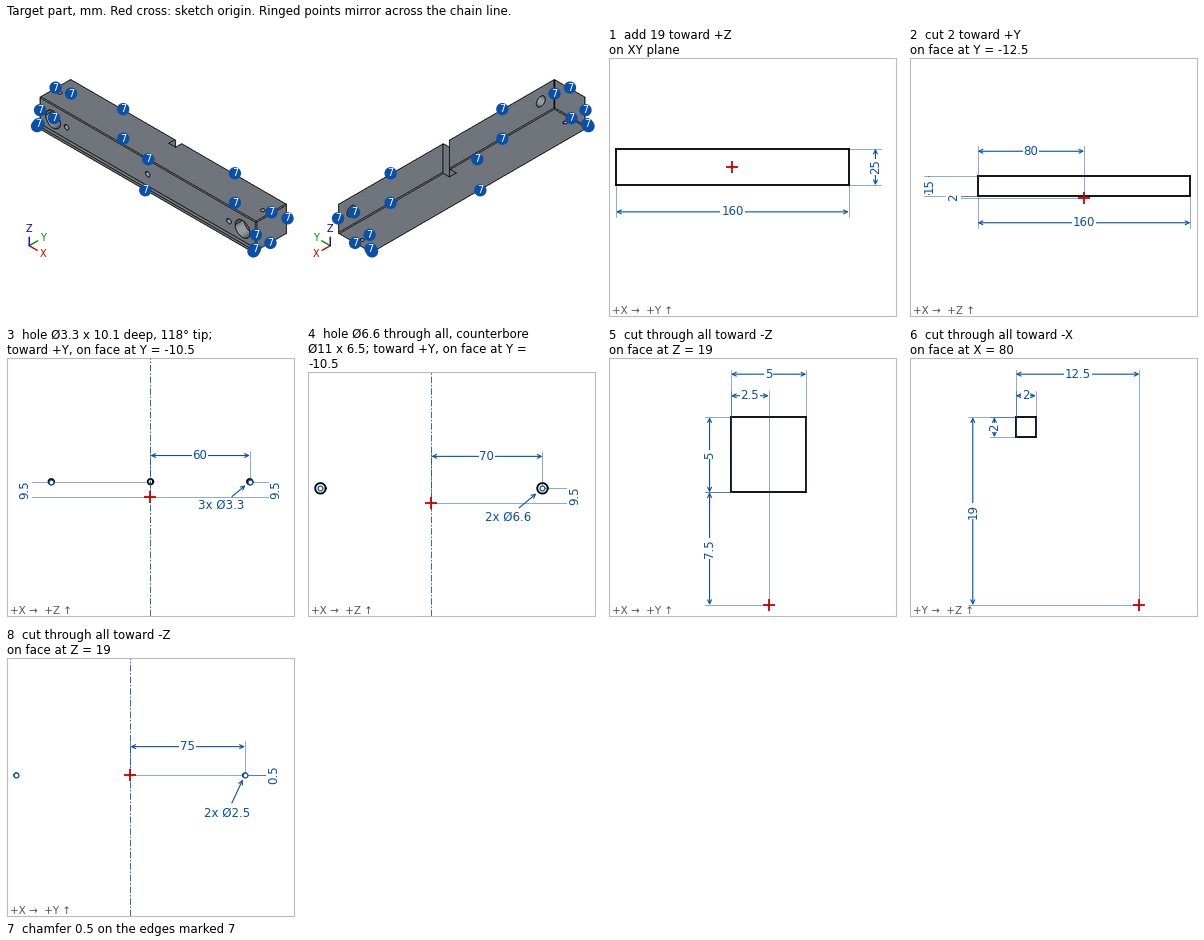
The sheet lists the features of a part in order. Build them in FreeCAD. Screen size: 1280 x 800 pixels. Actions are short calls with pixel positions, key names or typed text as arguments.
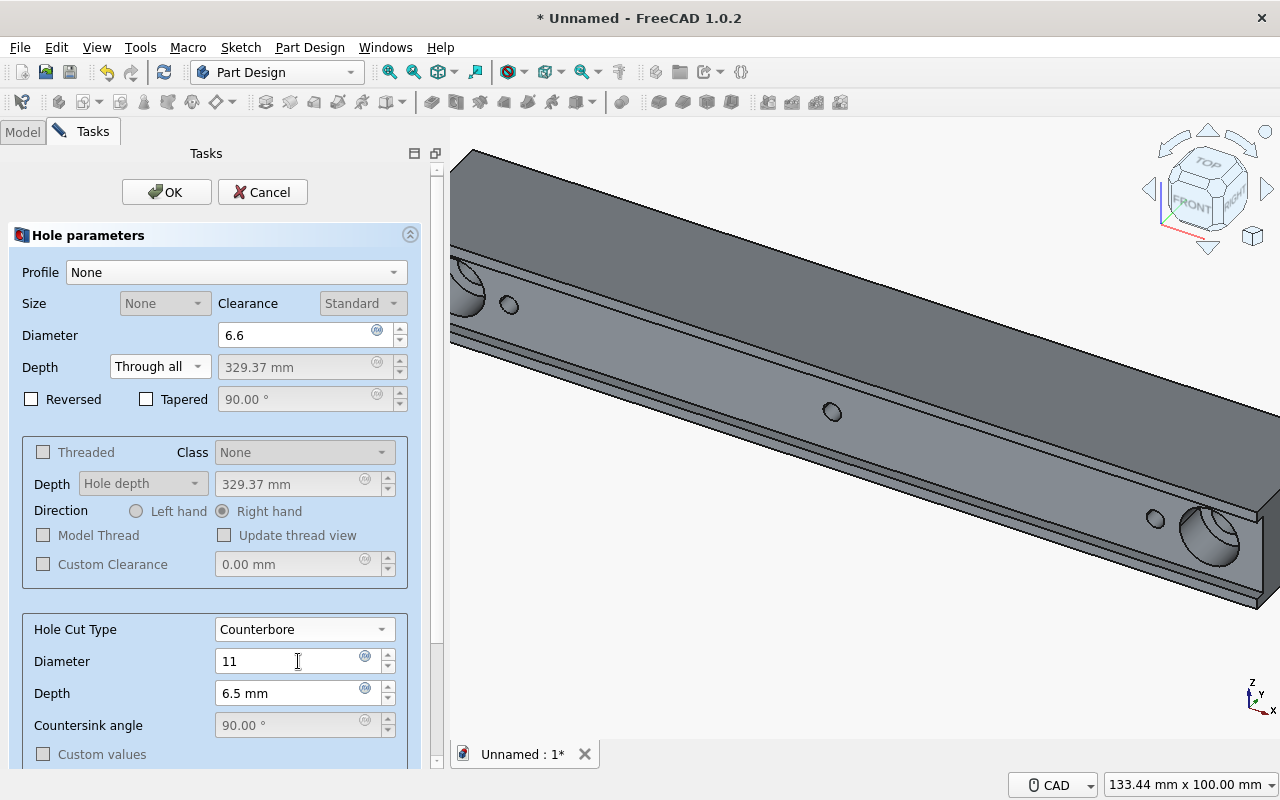
click(167, 192)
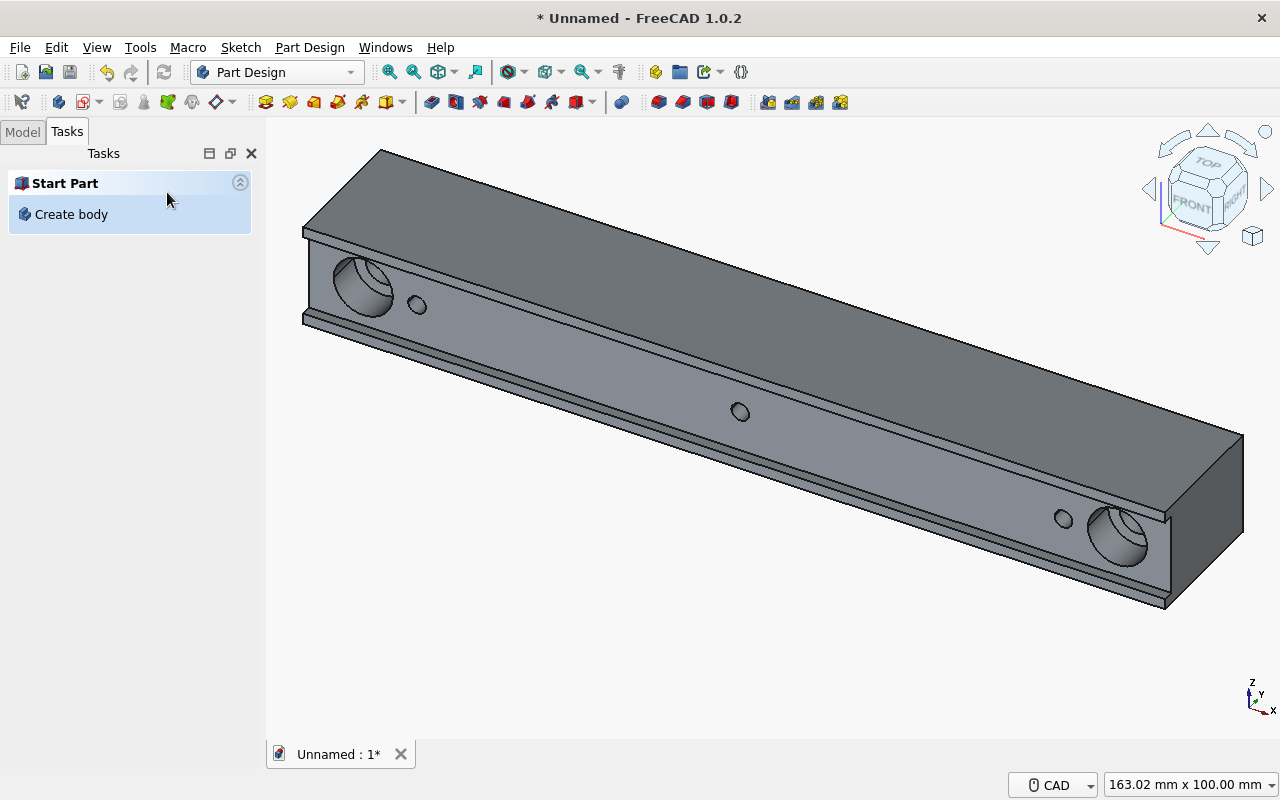
click(1019, 412)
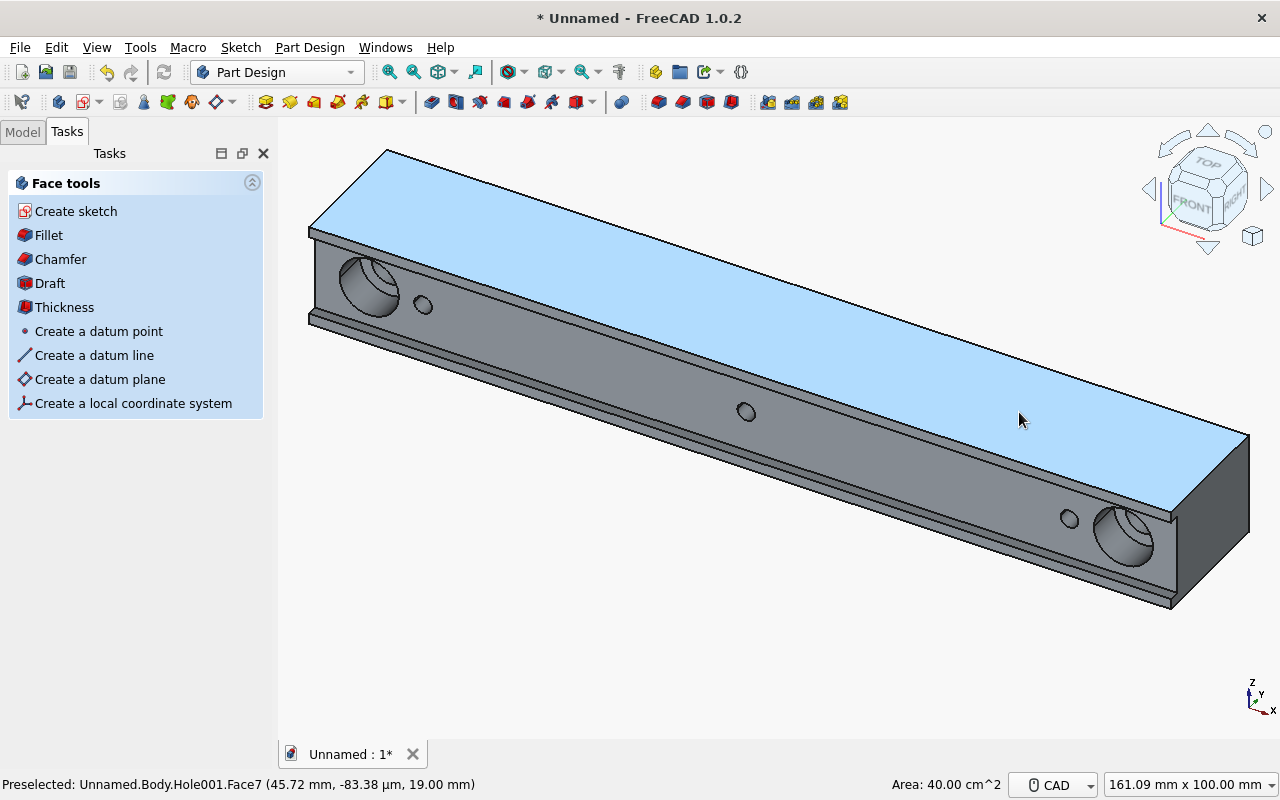
click(84, 102)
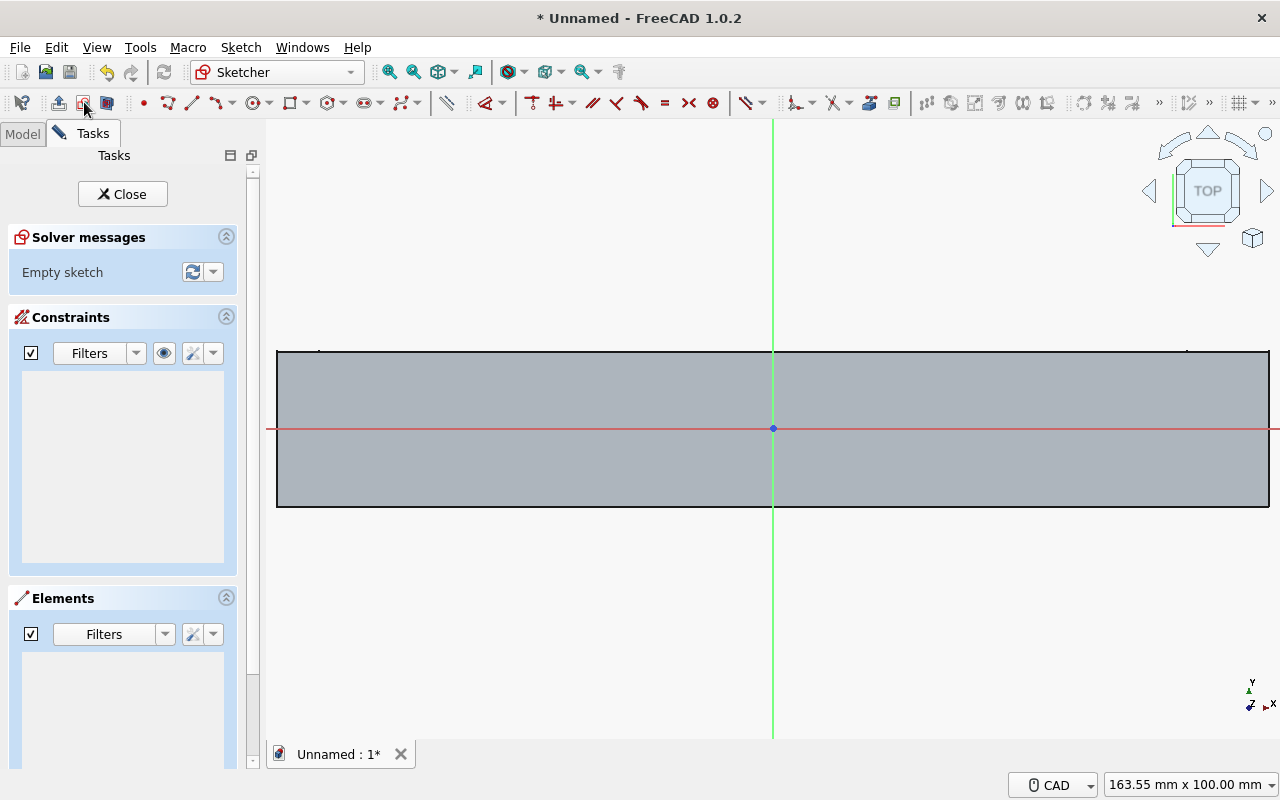
scroll(778, 362, up, 13)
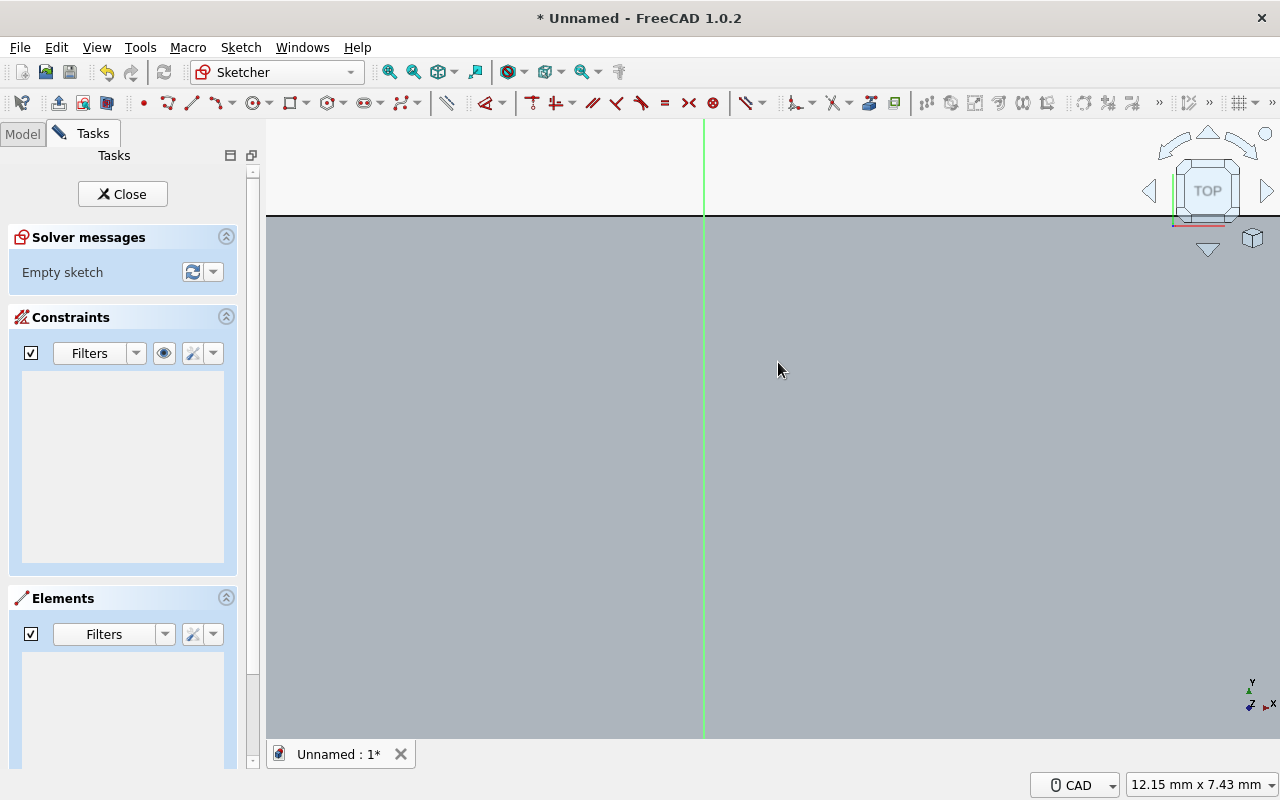
click(290, 104)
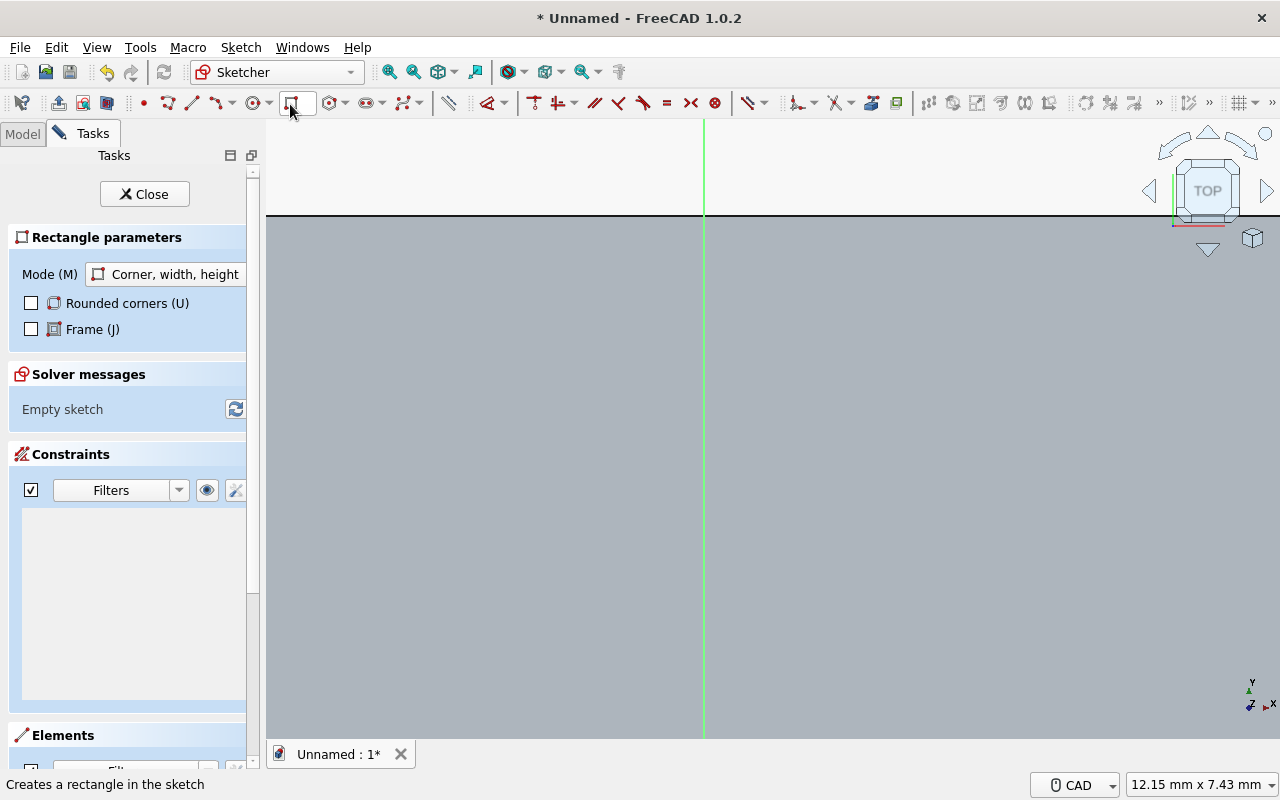
click(496, 216)
click(913, 633)
key(Escape)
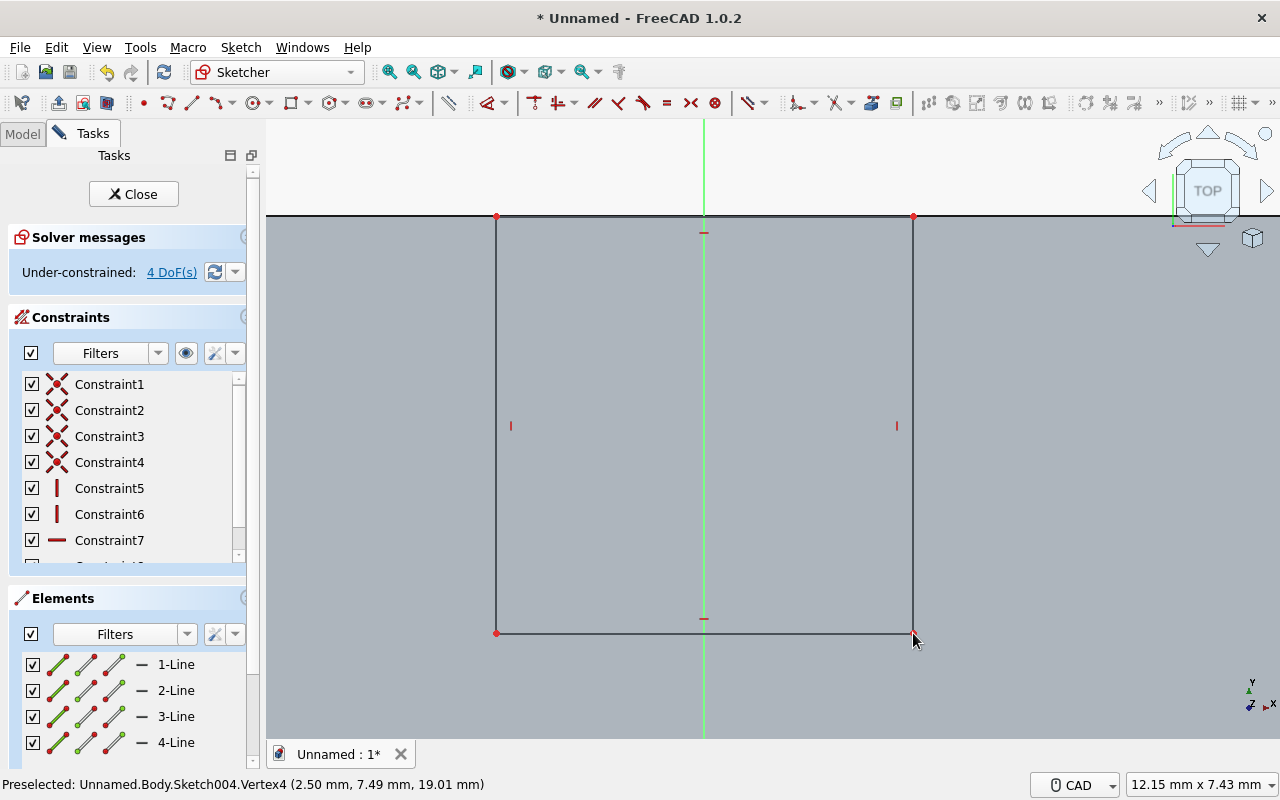
key(d)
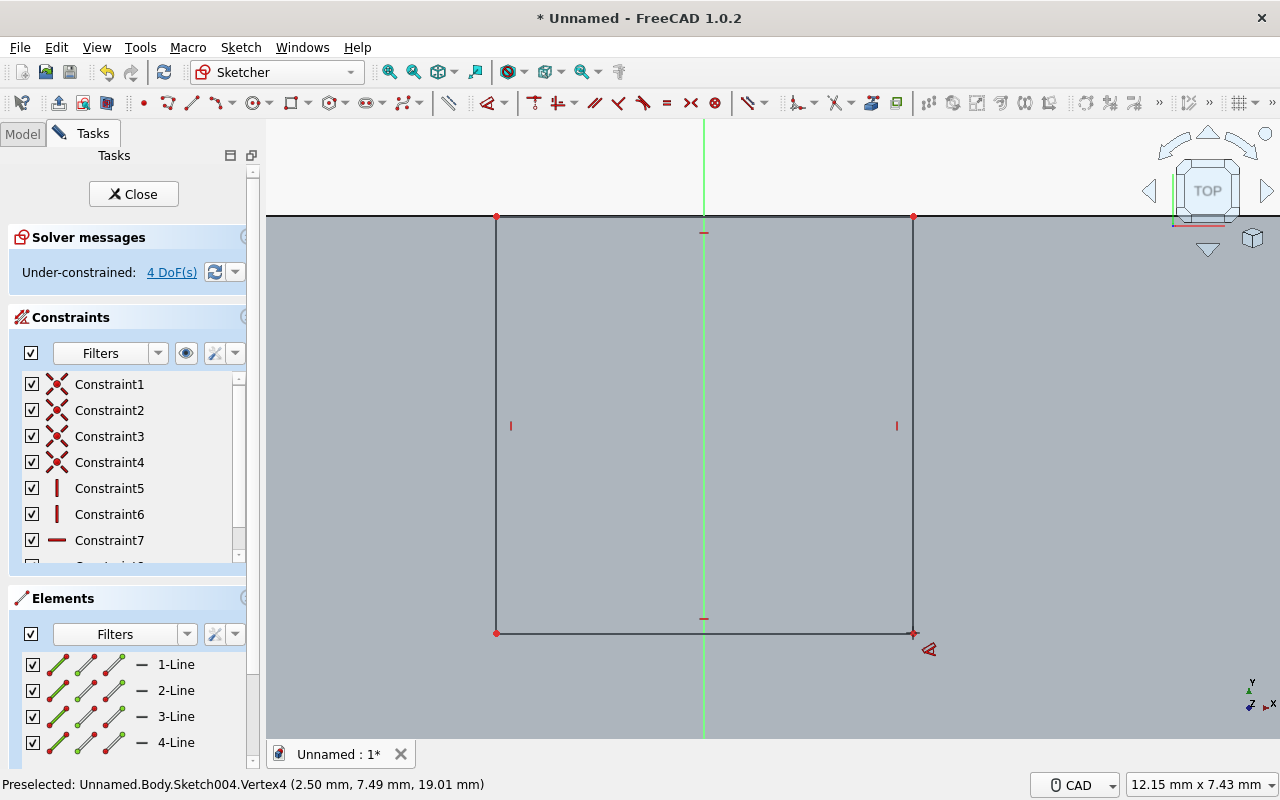
click(496, 342)
click(462, 426)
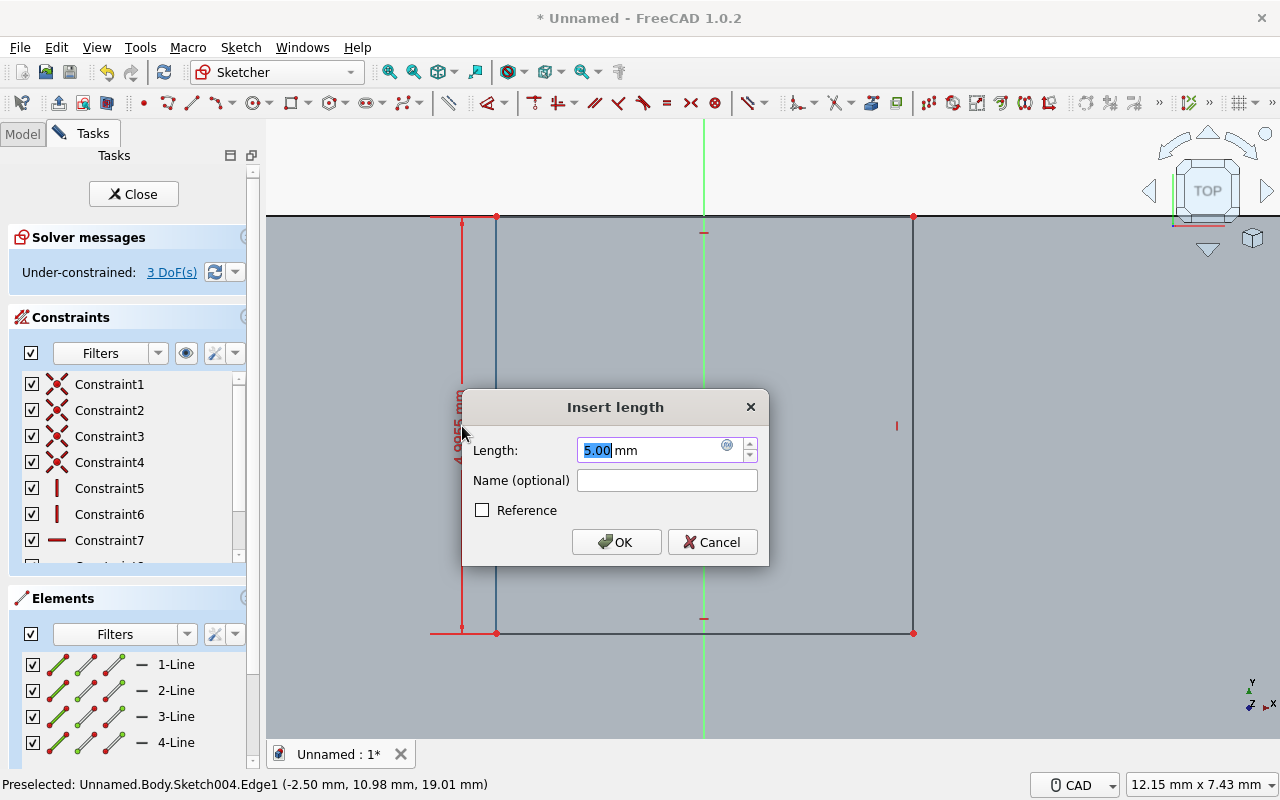
text(5)
key(Return)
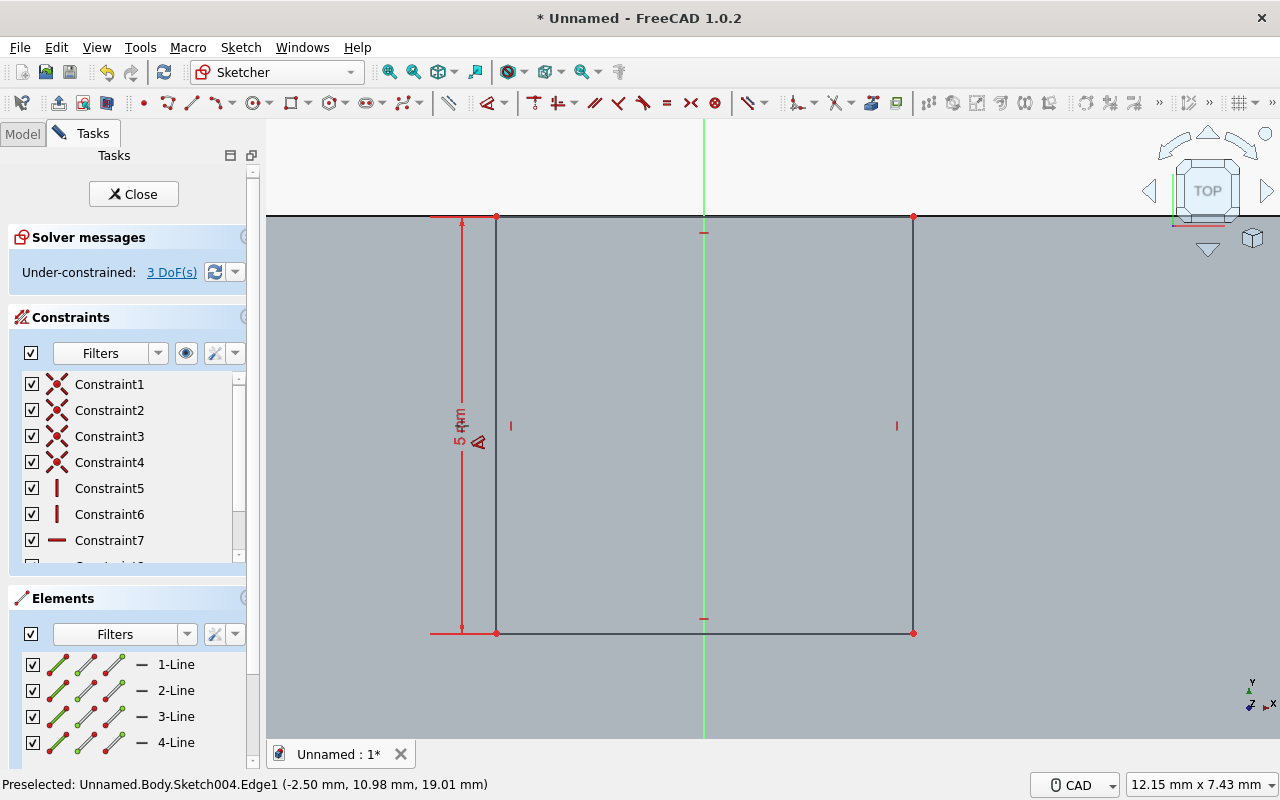
click(621, 634)
click(609, 668)